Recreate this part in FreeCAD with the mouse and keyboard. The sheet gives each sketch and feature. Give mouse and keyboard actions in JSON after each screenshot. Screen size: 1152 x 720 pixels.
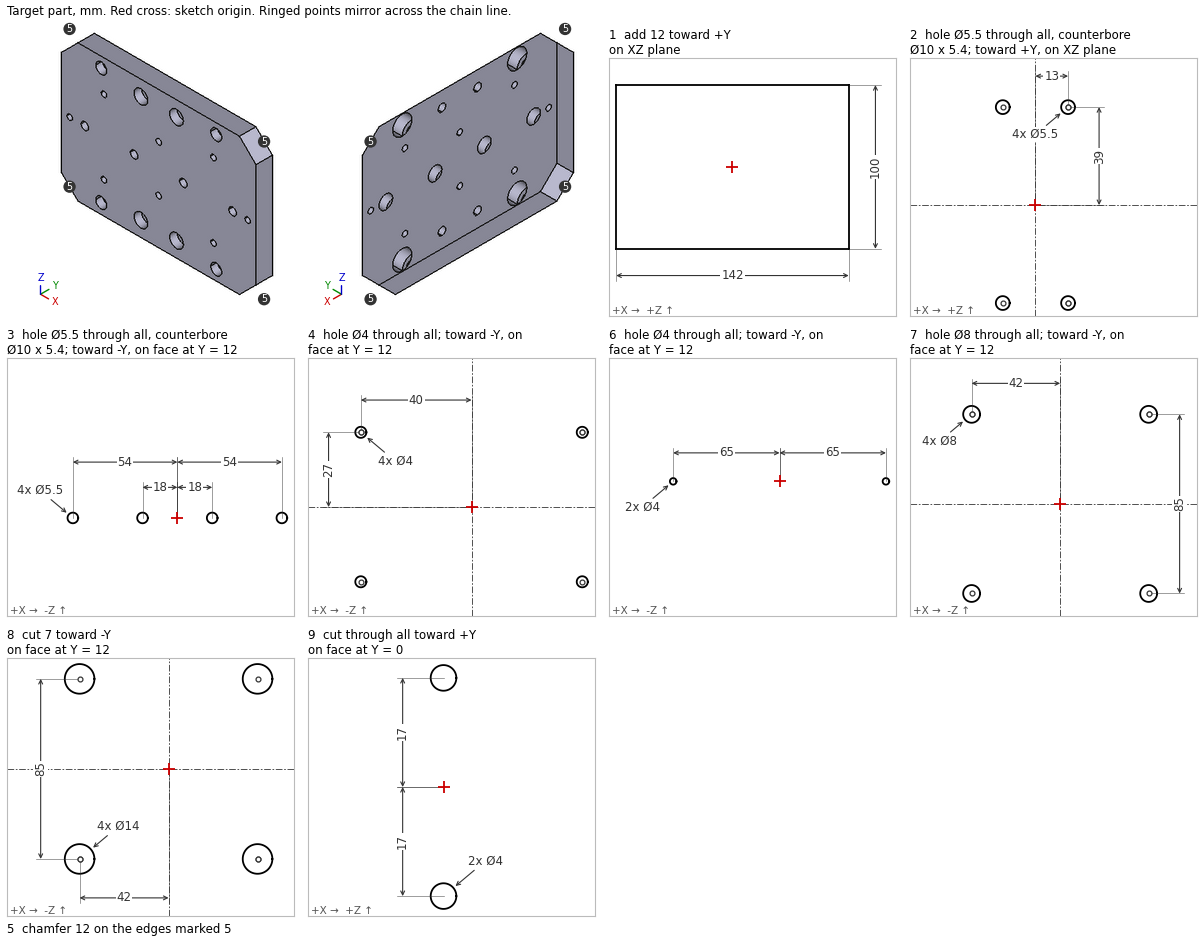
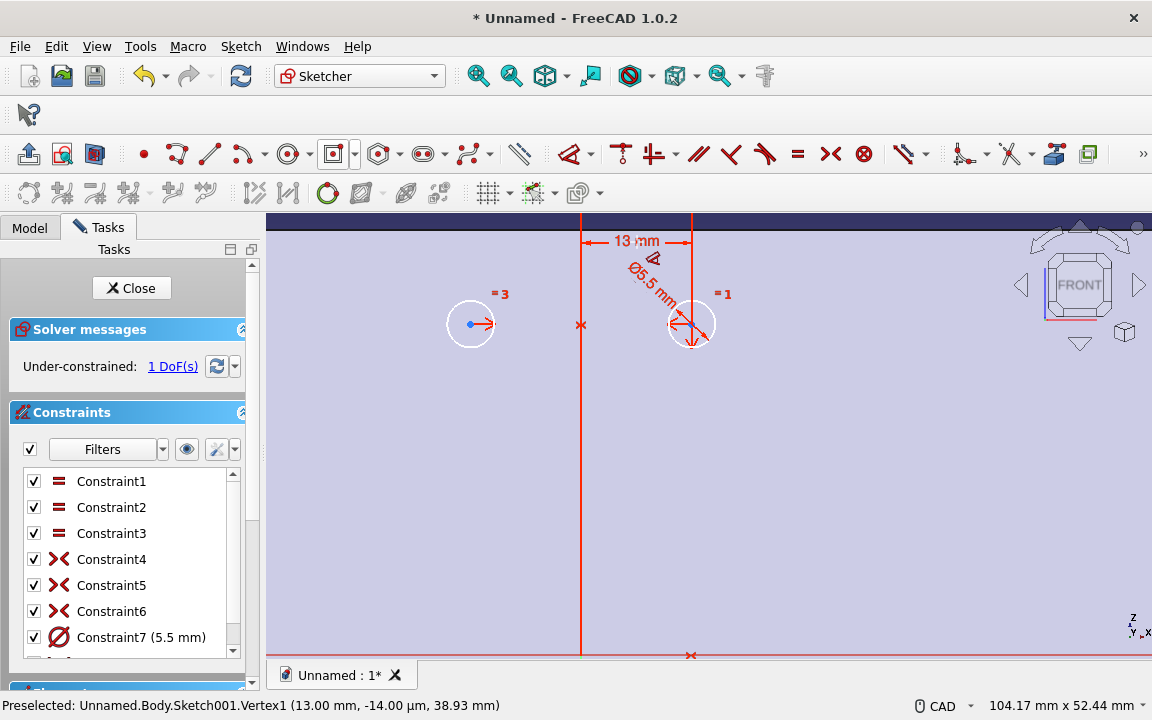
{"action": "left_click", "coordinate": [692, 324]}
{"action": "left_click", "coordinate": [726, 478]}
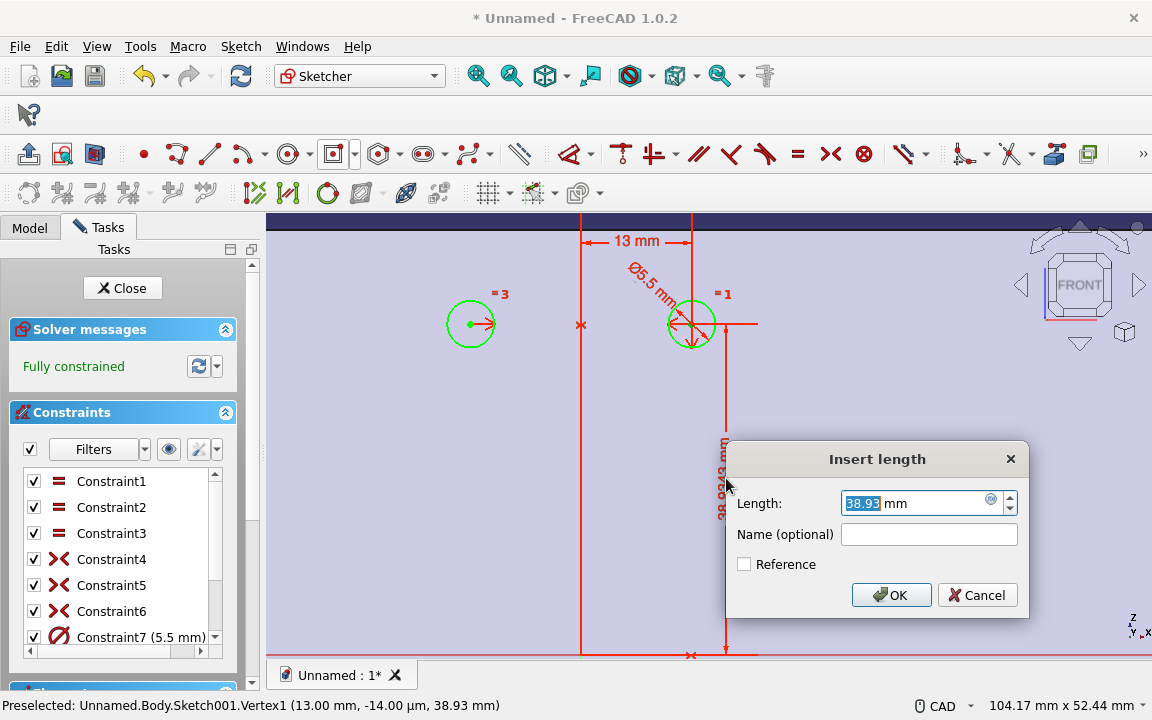
{"action": "type", "text": "39"}
{"action": "key", "text": "Return"}
{"action": "key", "text": "Escape"}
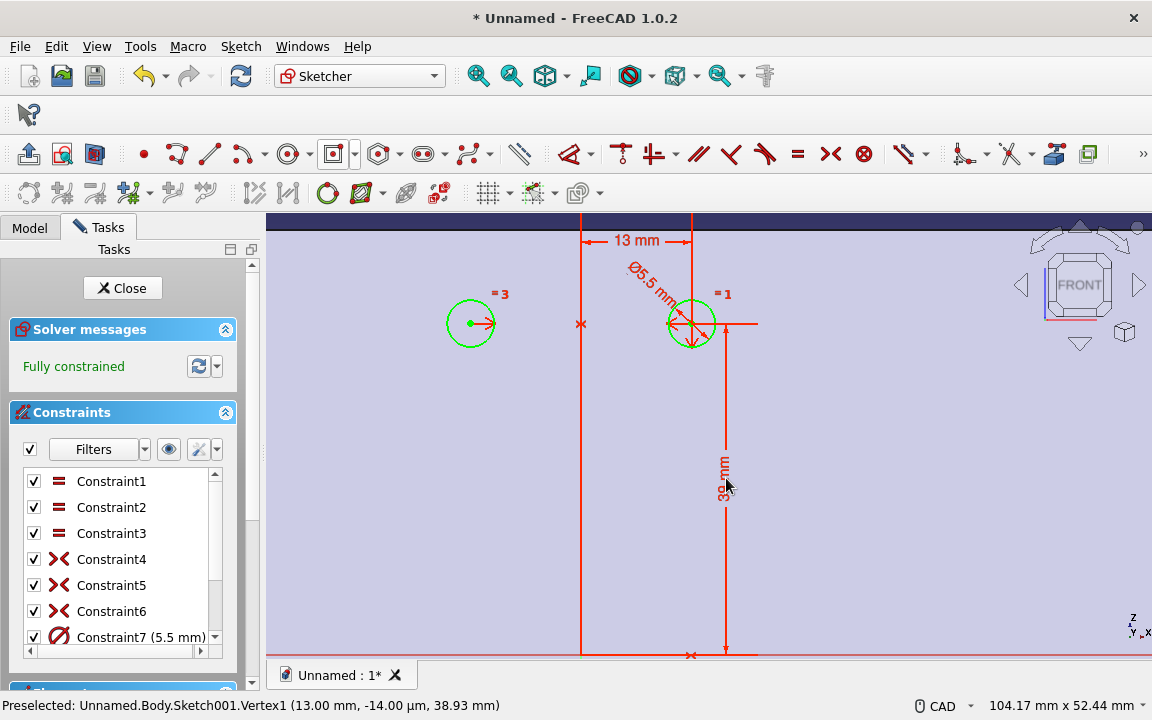
{"action": "left_click", "coordinate": [123, 288]}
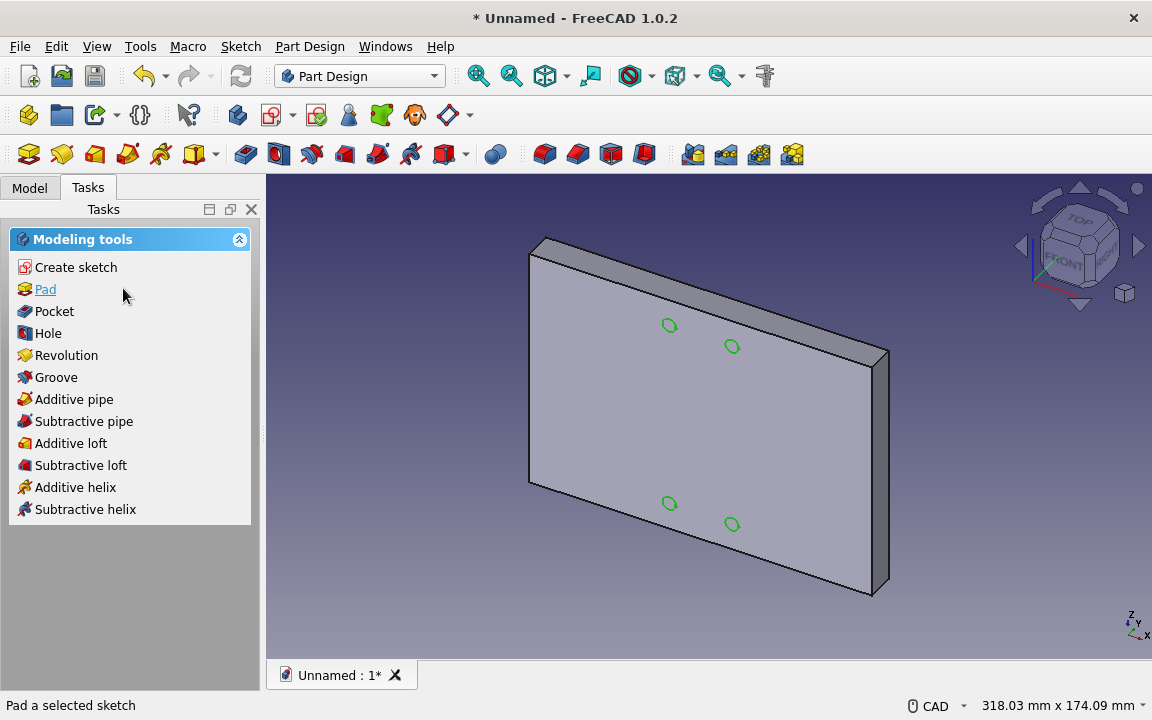
{"action": "left_click", "coordinate": [279, 154]}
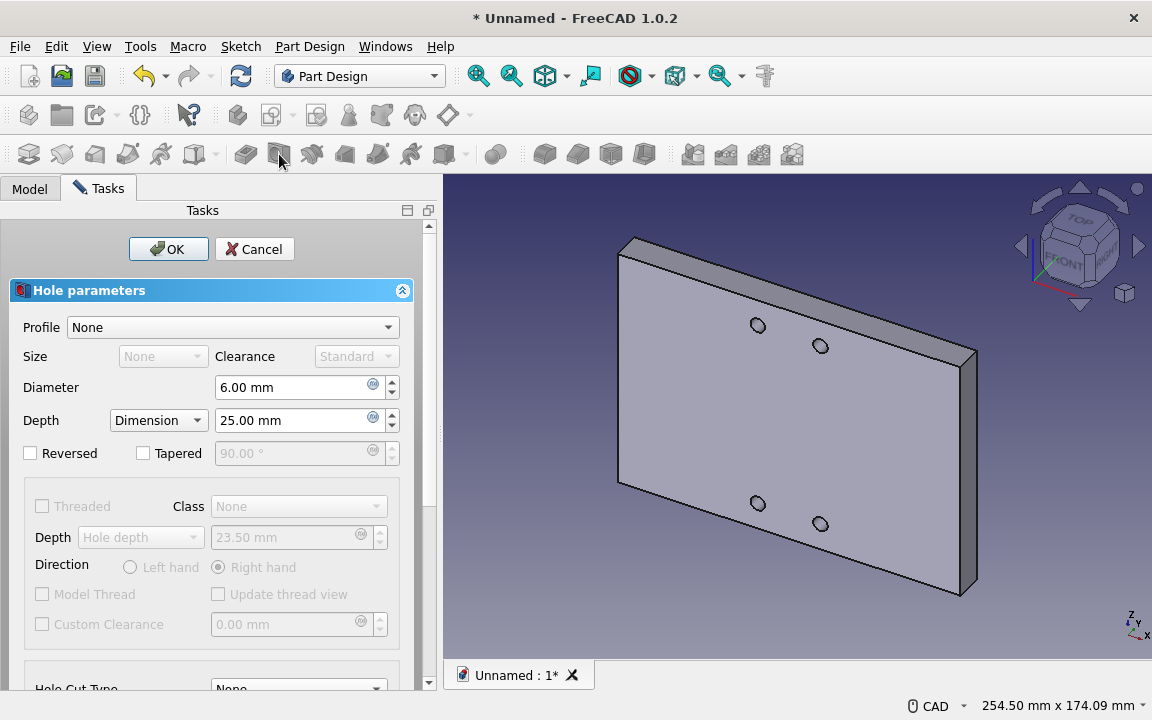
{"action": "triple_click", "coordinate": [300, 388]}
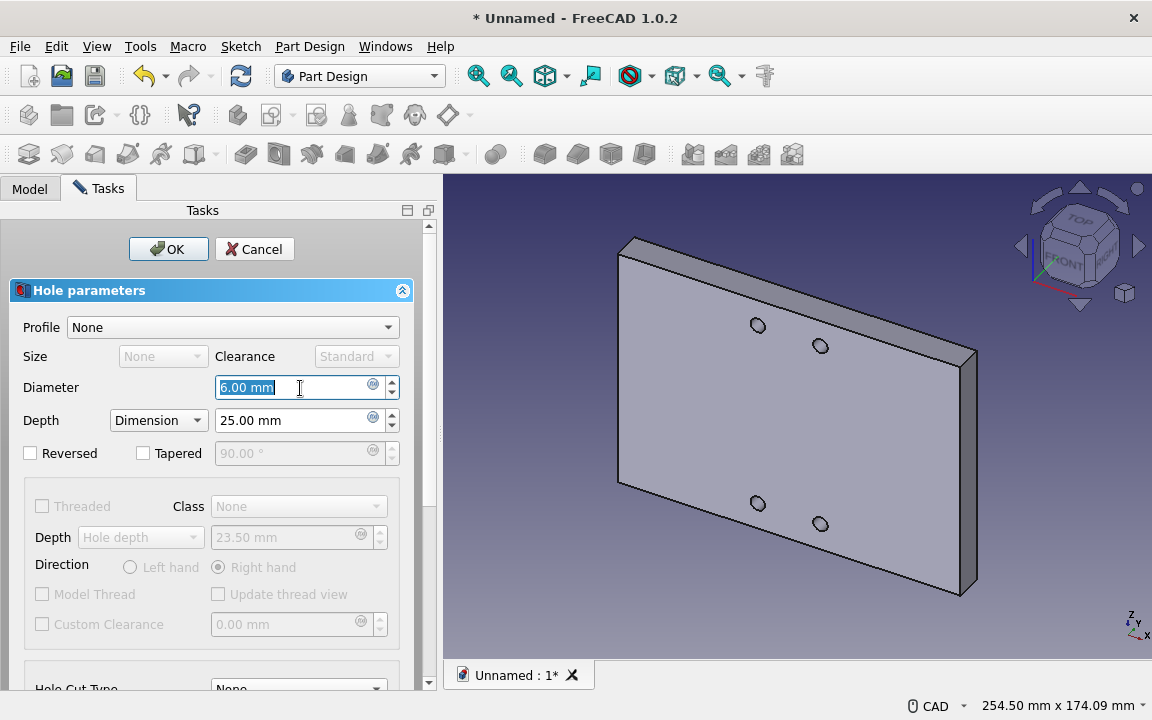
{"action": "type", "text": "5.5"}
{"action": "key", "text": "Tab"}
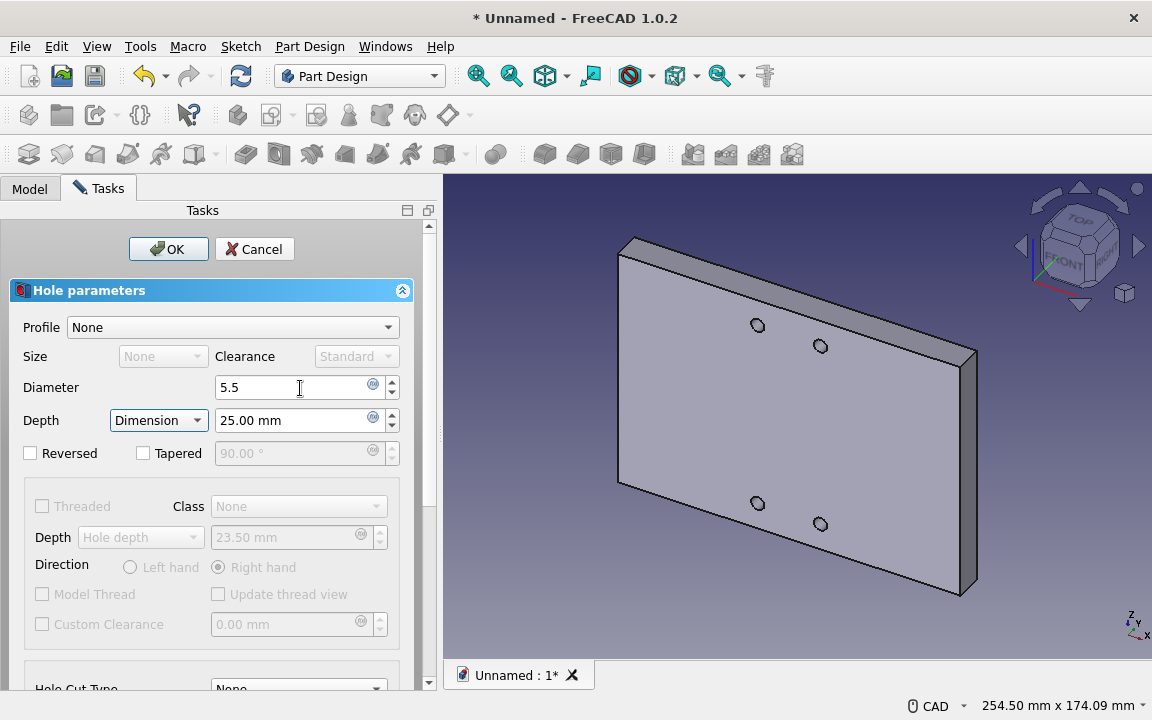
{"action": "left_click", "coordinate": [160, 420]}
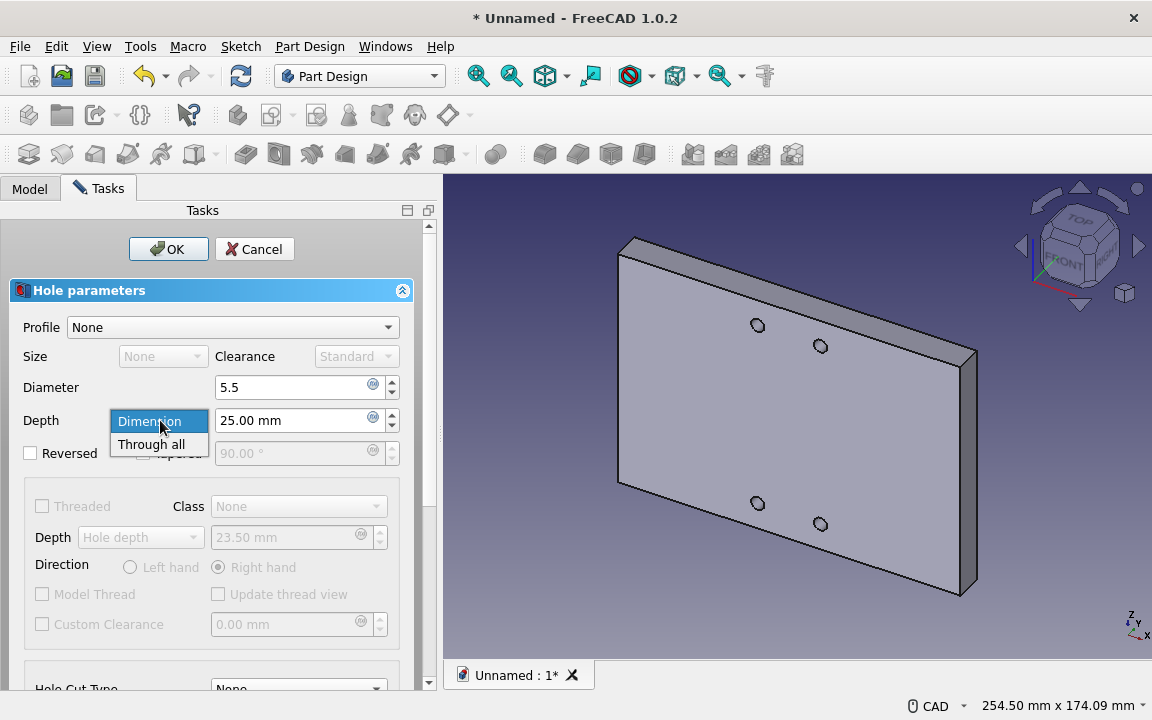
{"action": "left_click", "coordinate": [158, 444]}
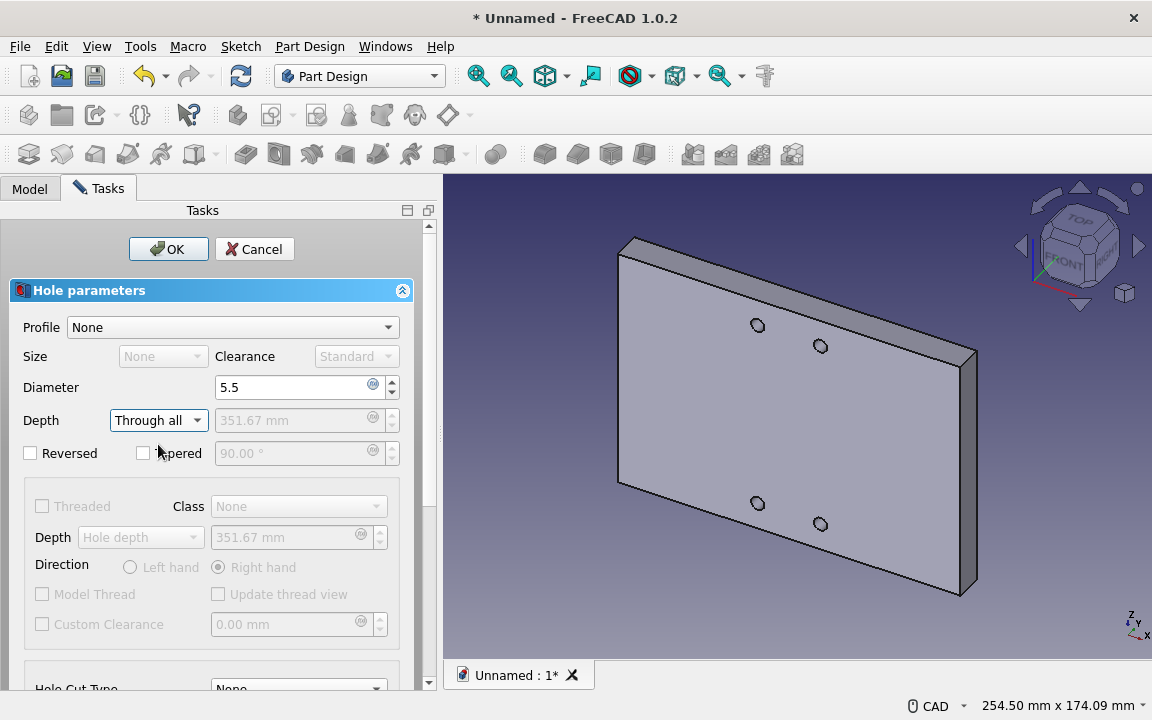
{"action": "scroll", "coordinate": [429, 455], "scroll_direction": "down", "scroll_amount": 2}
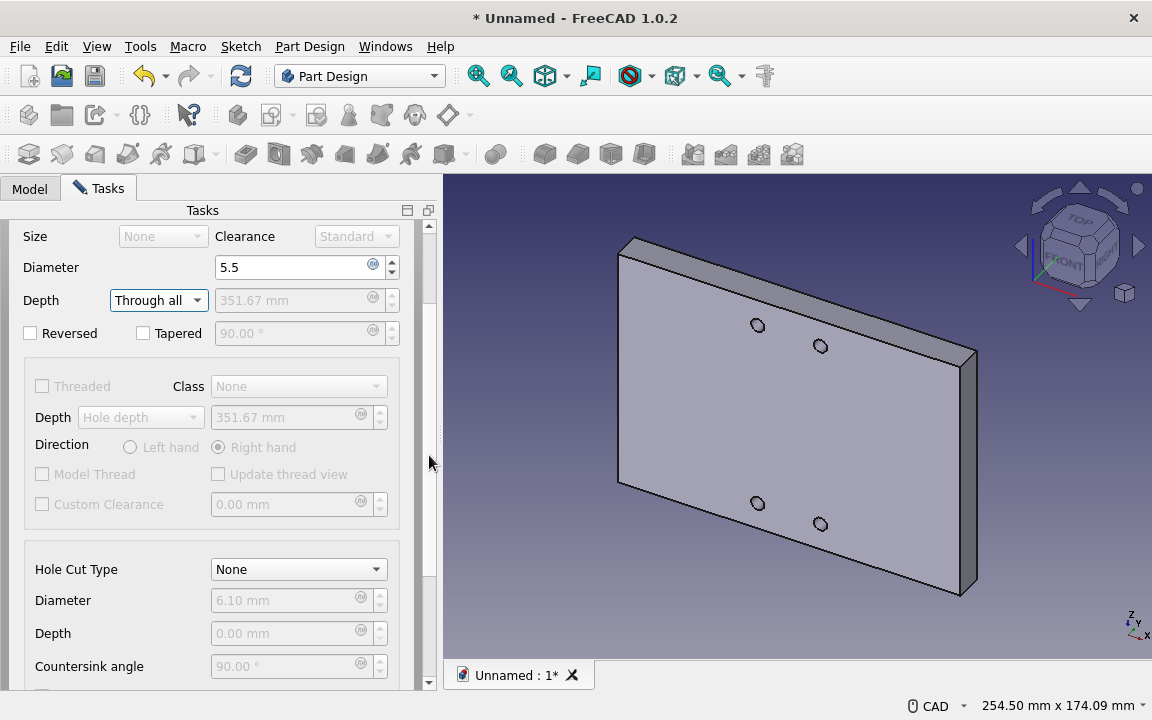
{"action": "left_click", "coordinate": [300, 570]}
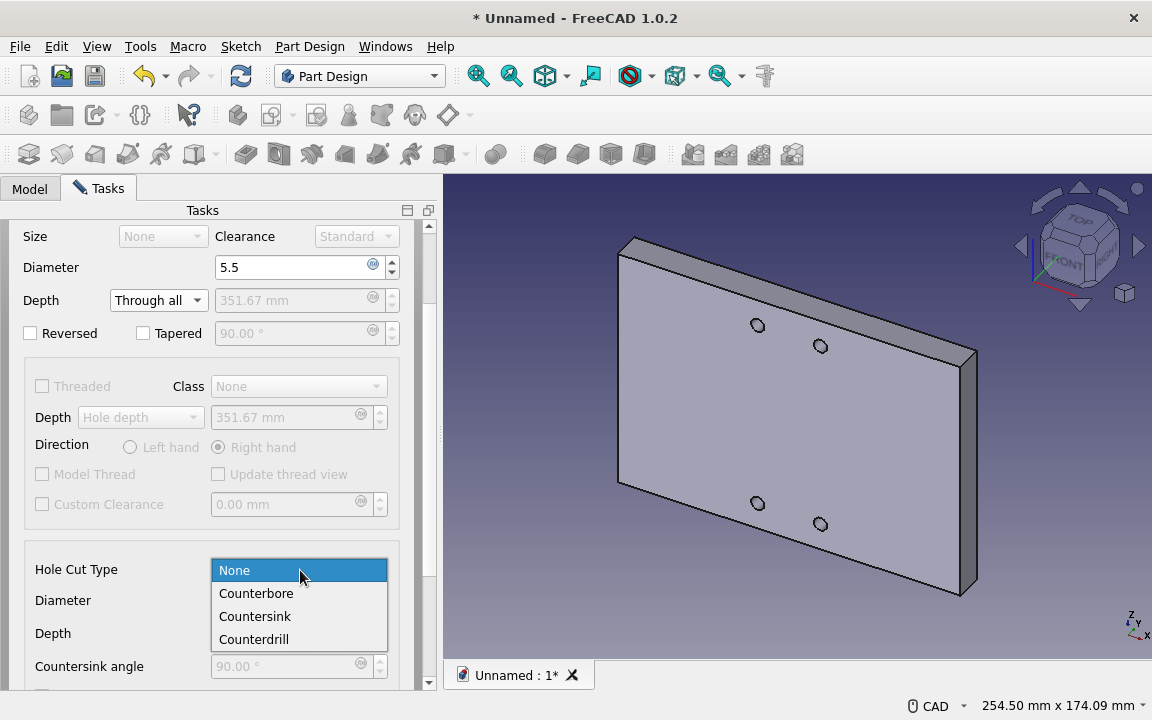
{"action": "left_click", "coordinate": [298, 594]}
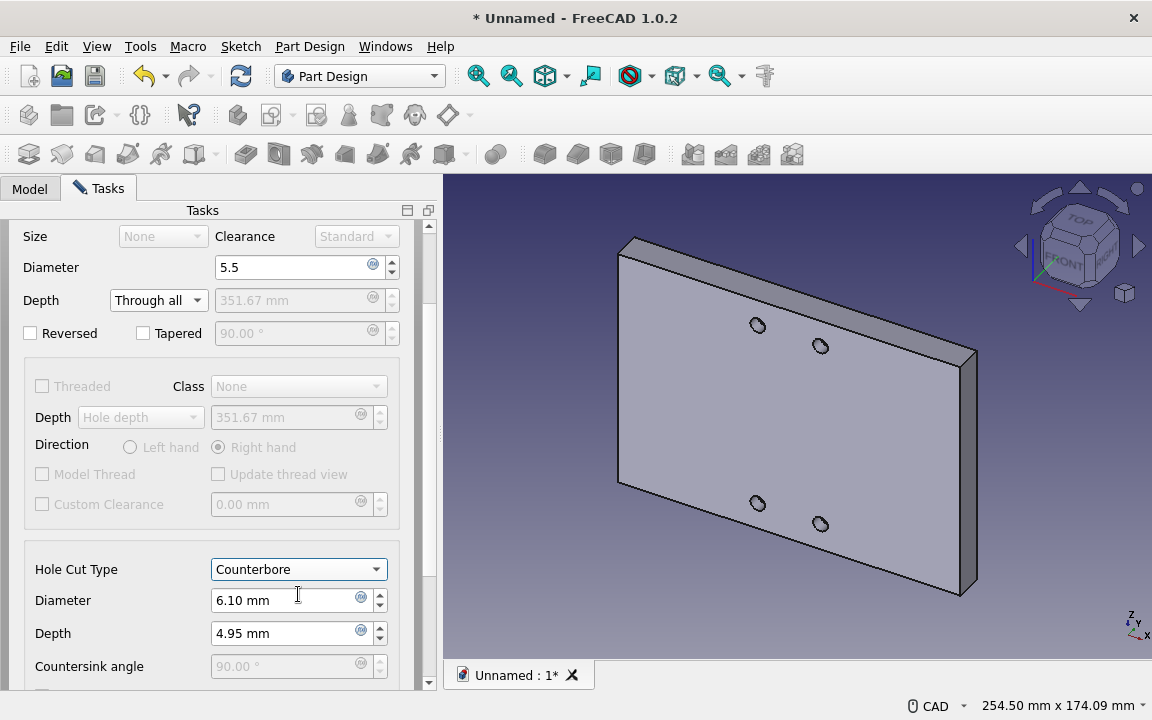
{"action": "triple_click", "coordinate": [292, 600]}